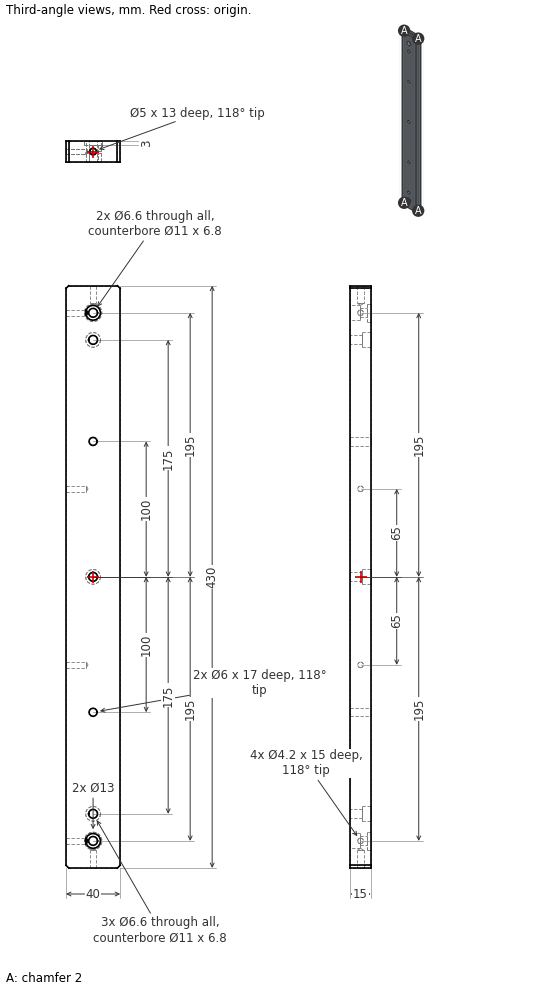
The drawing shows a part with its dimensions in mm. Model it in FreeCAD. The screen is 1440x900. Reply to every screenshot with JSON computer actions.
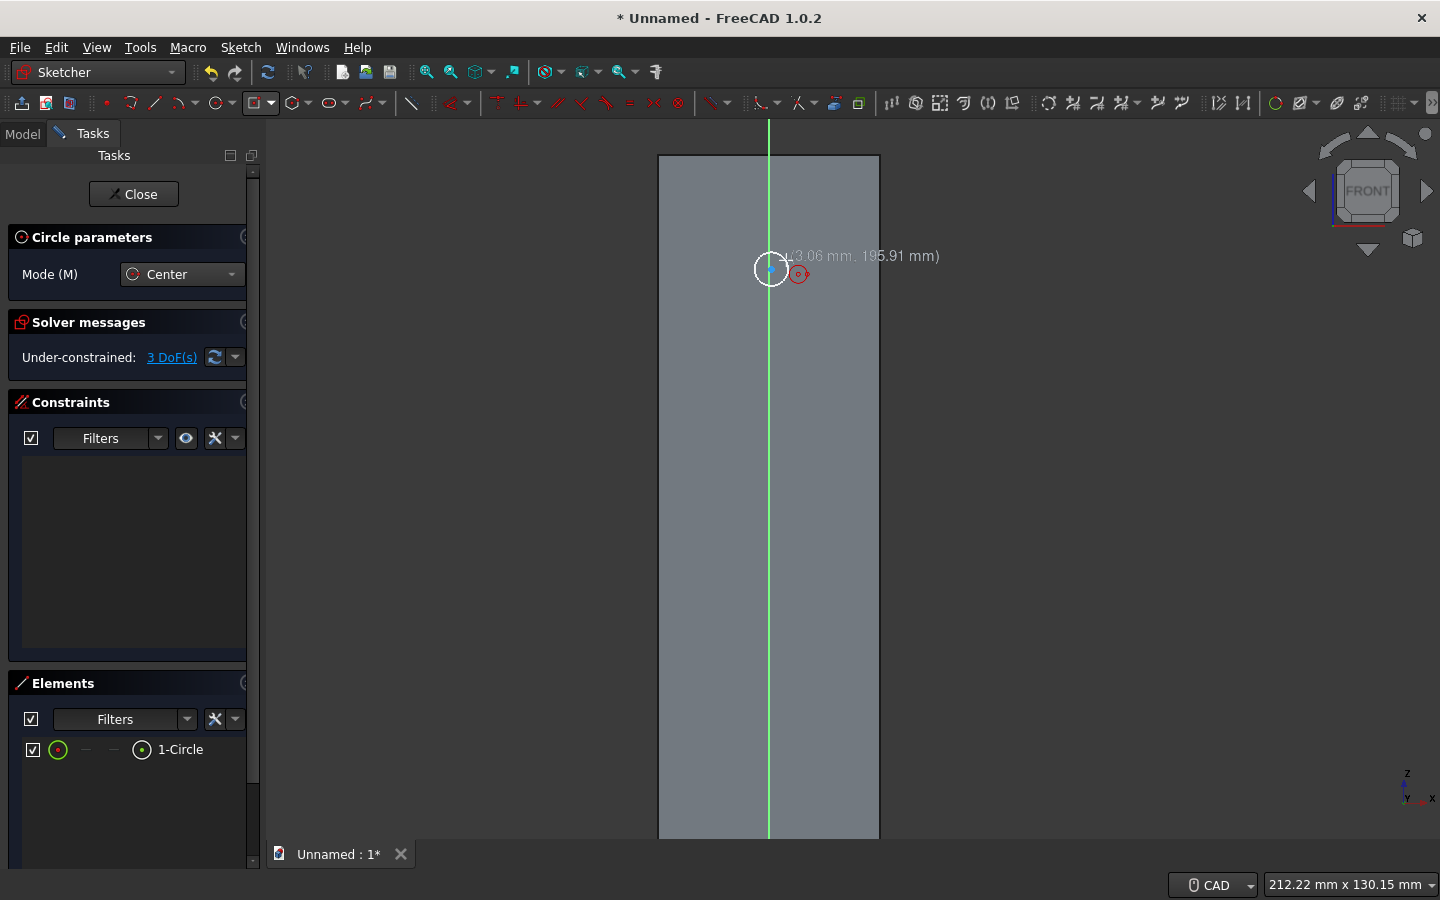
{"action": "scroll", "coordinate": [788, 260], "scroll_direction": "down", "scroll_amount": 8}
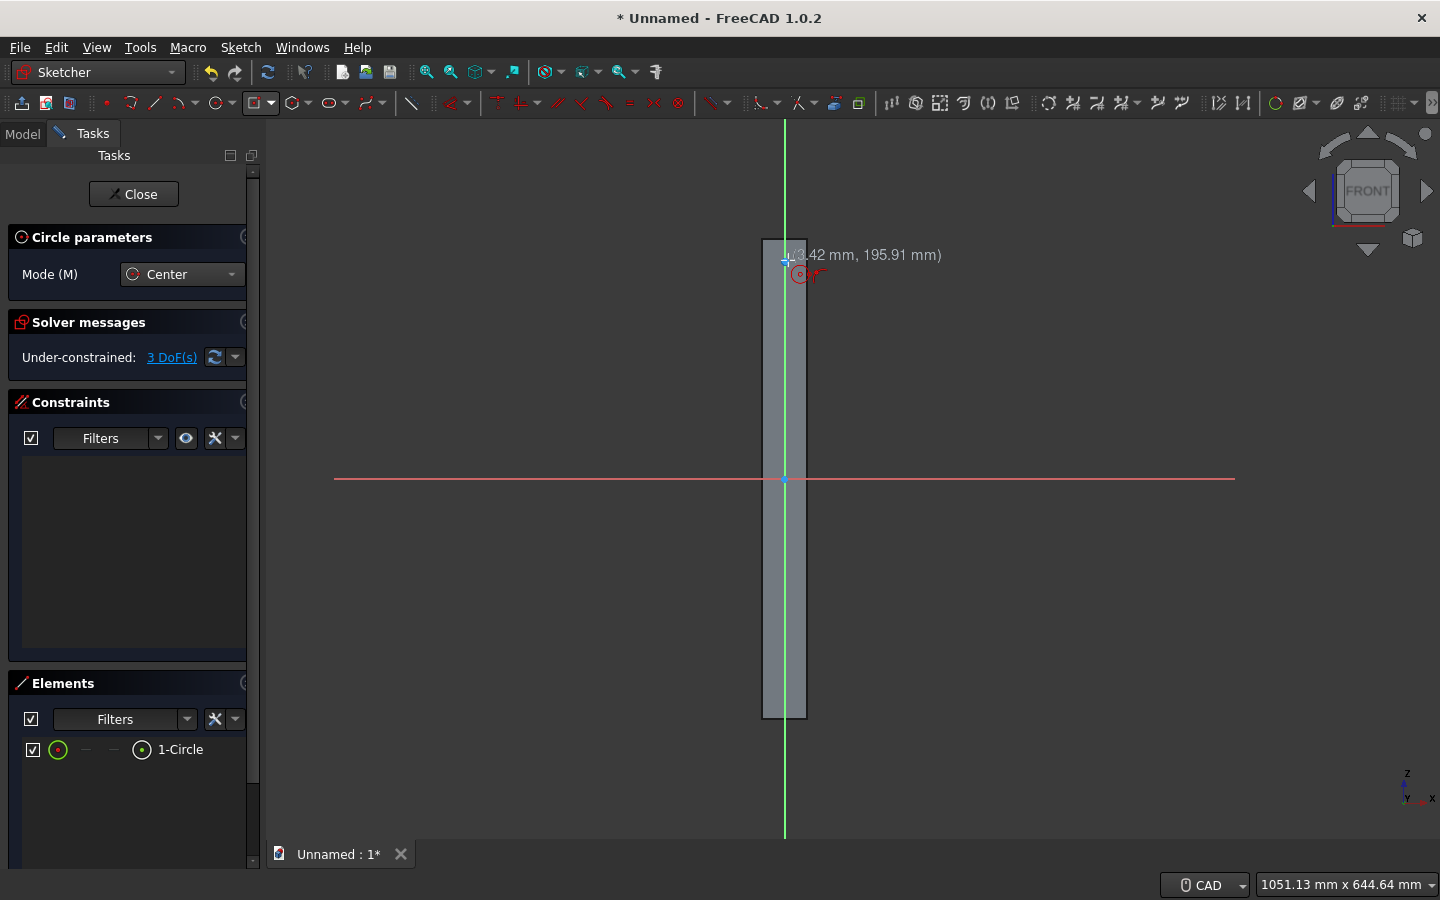
{"action": "scroll", "coordinate": [785, 697], "scroll_direction": "up", "scroll_amount": 10}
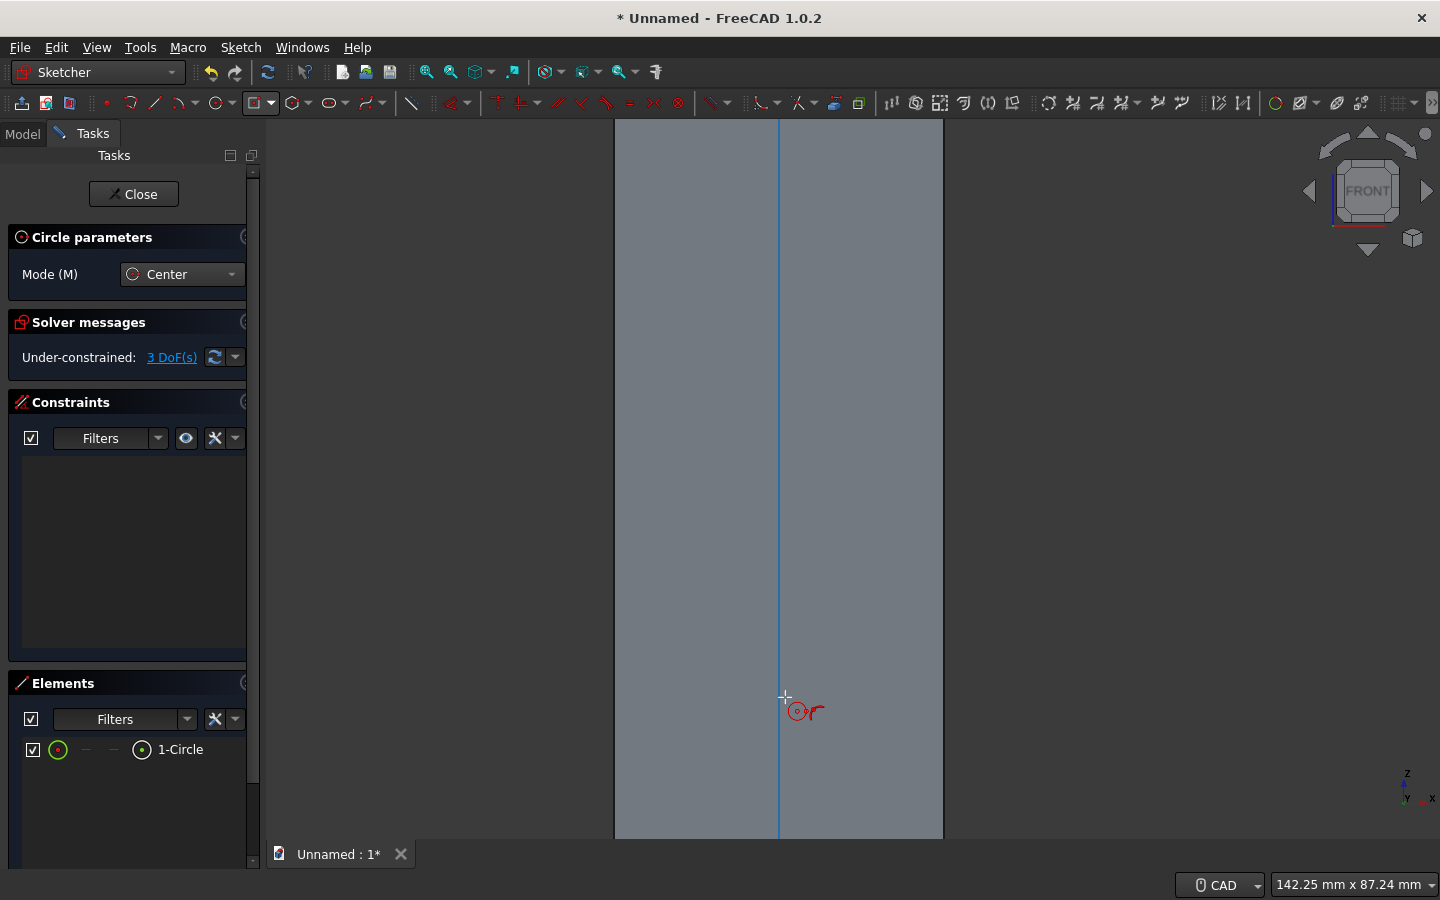
{"action": "scroll", "coordinate": [785, 698], "scroll_direction": "down", "scroll_amount": 10}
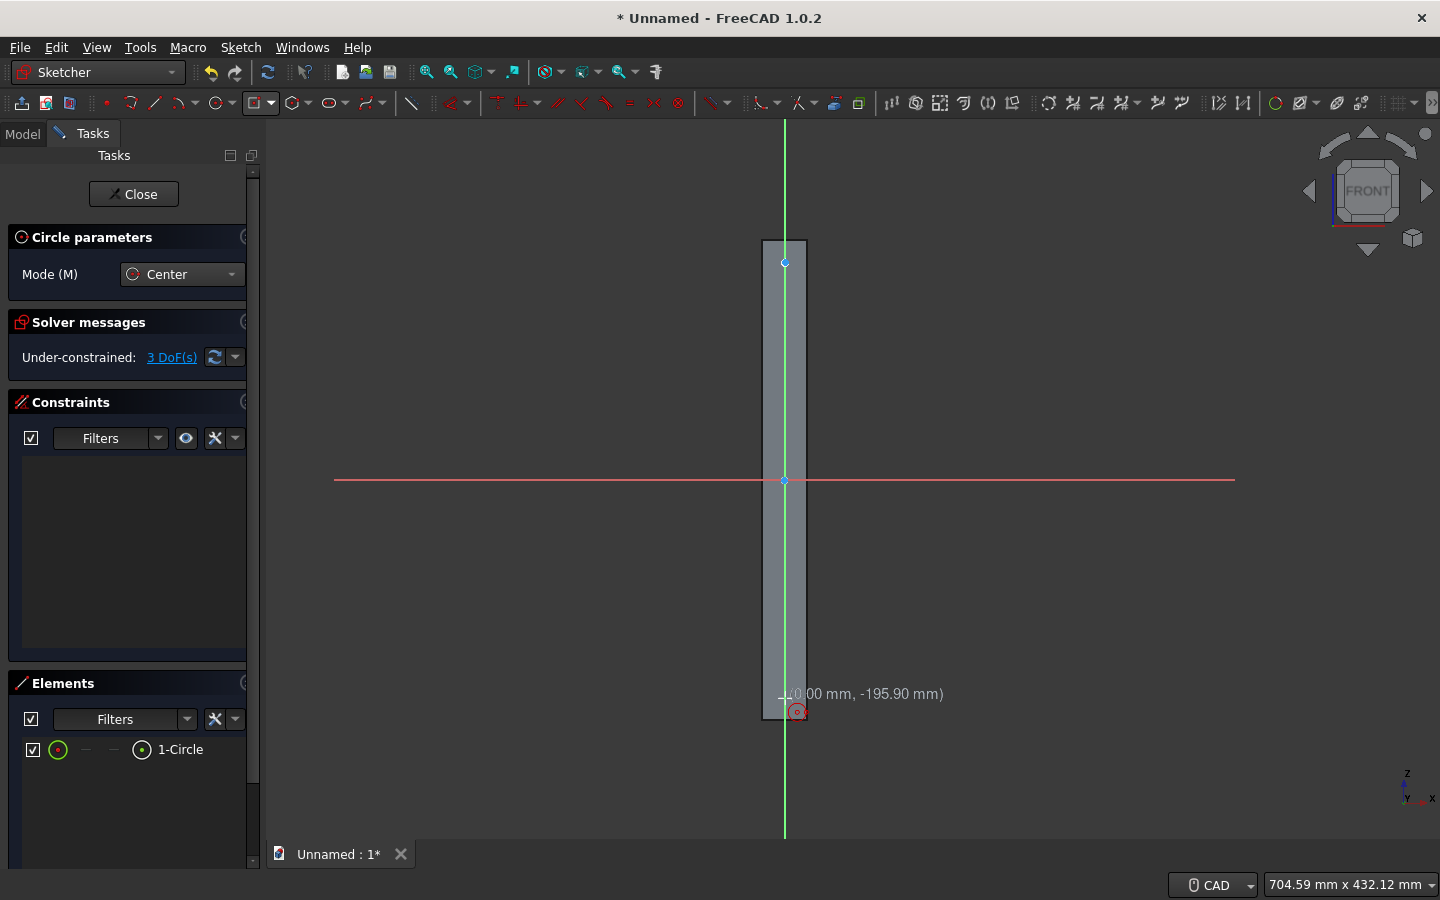
{"action": "left_click", "coordinate": [785, 698]}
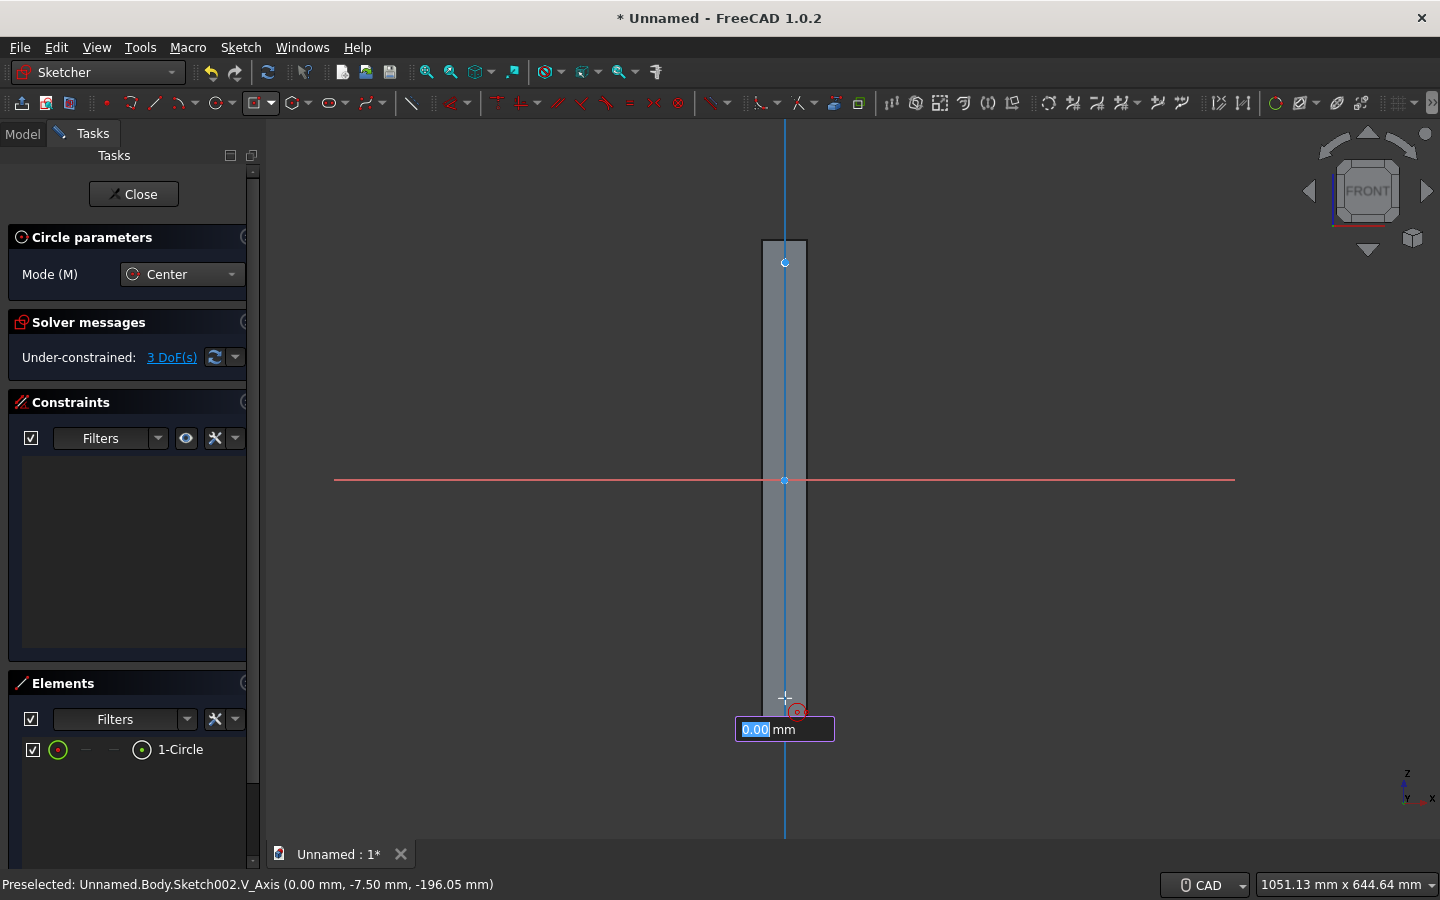
{"action": "scroll", "coordinate": [788, 697], "scroll_direction": "up", "scroll_amount": 8}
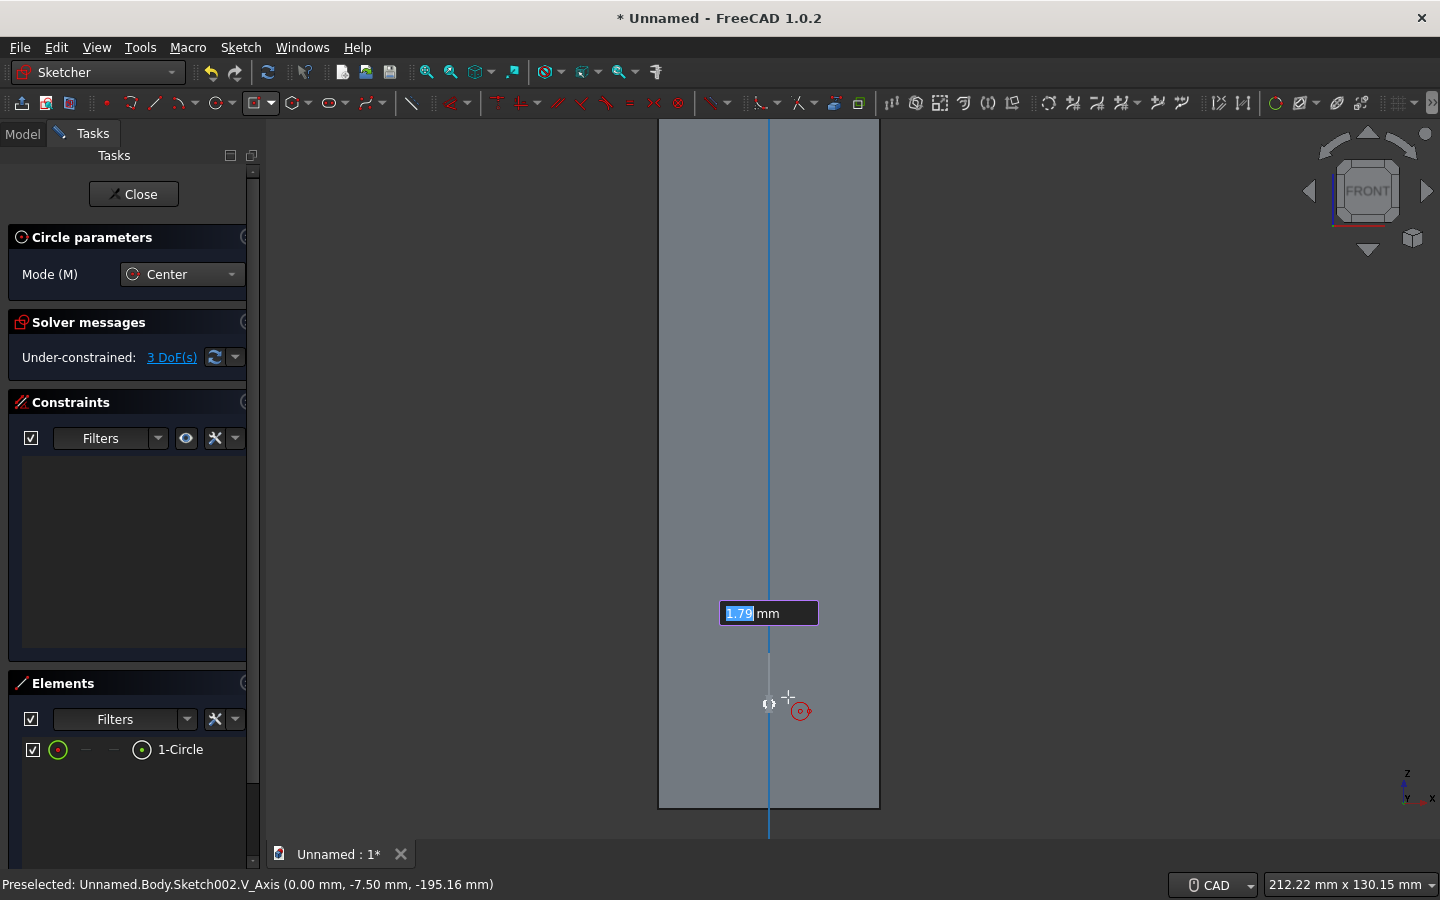
{"action": "left_click", "coordinate": [786, 692]}
{"action": "key", "text": "Escape"}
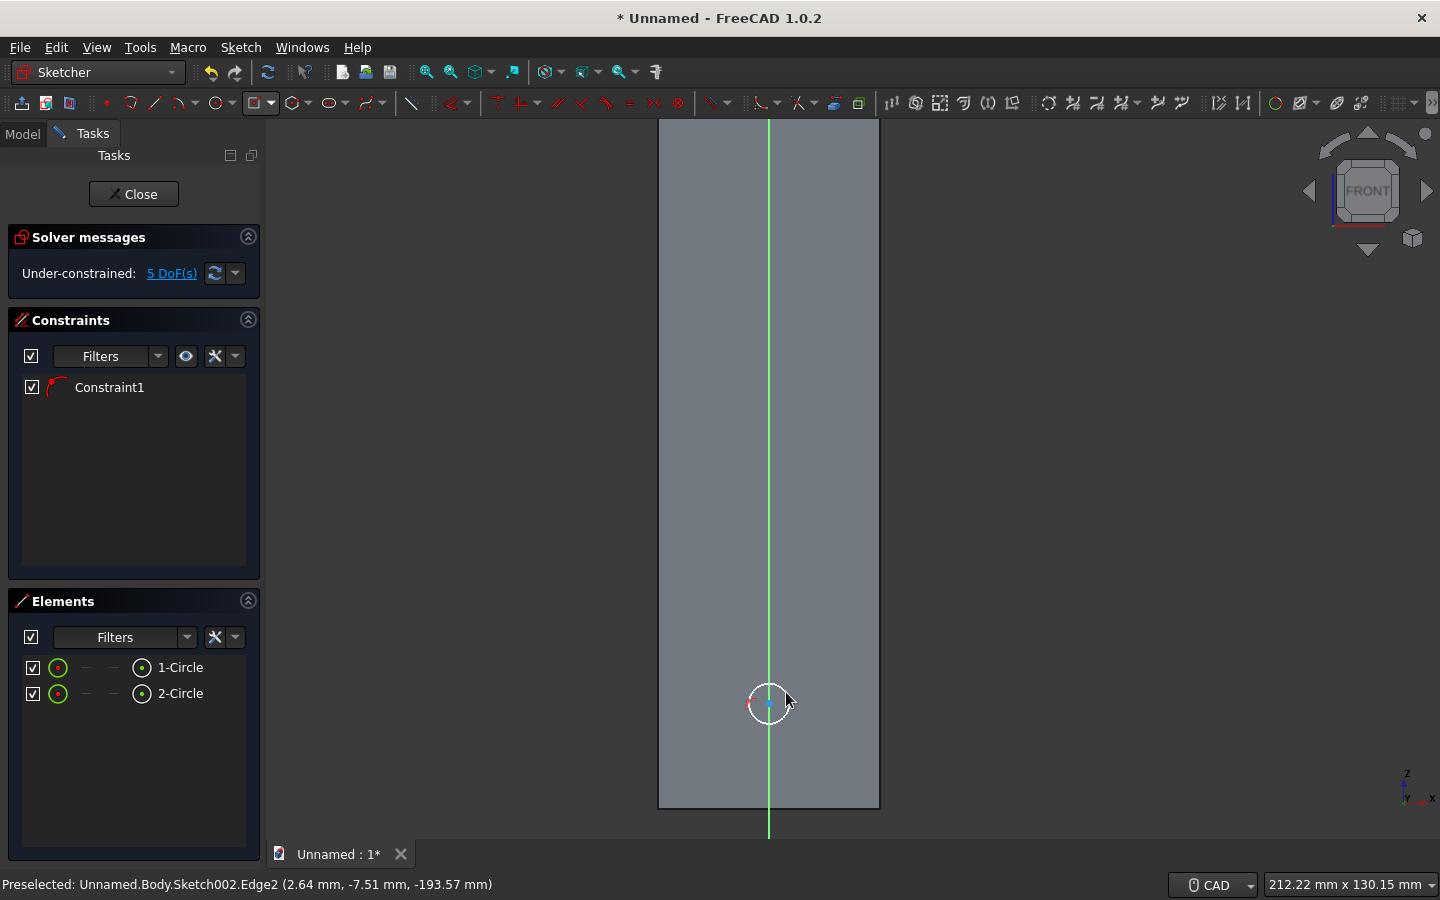
{"action": "scroll", "coordinate": [788, 697], "scroll_direction": "down", "scroll_amount": 8}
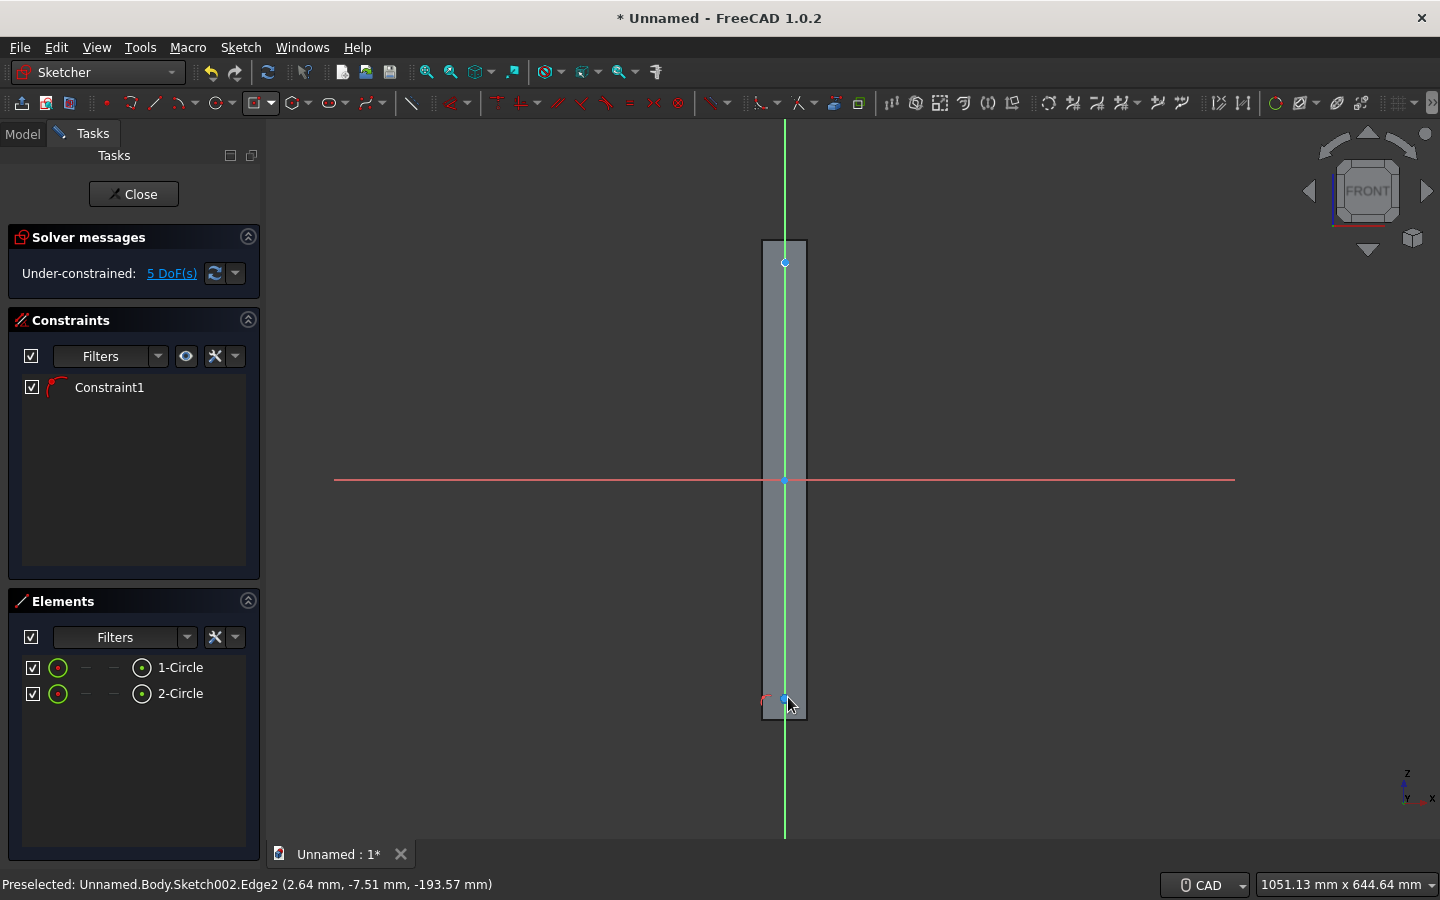
{"action": "scroll", "coordinate": [787, 260], "scroll_direction": "up", "scroll_amount": 8}